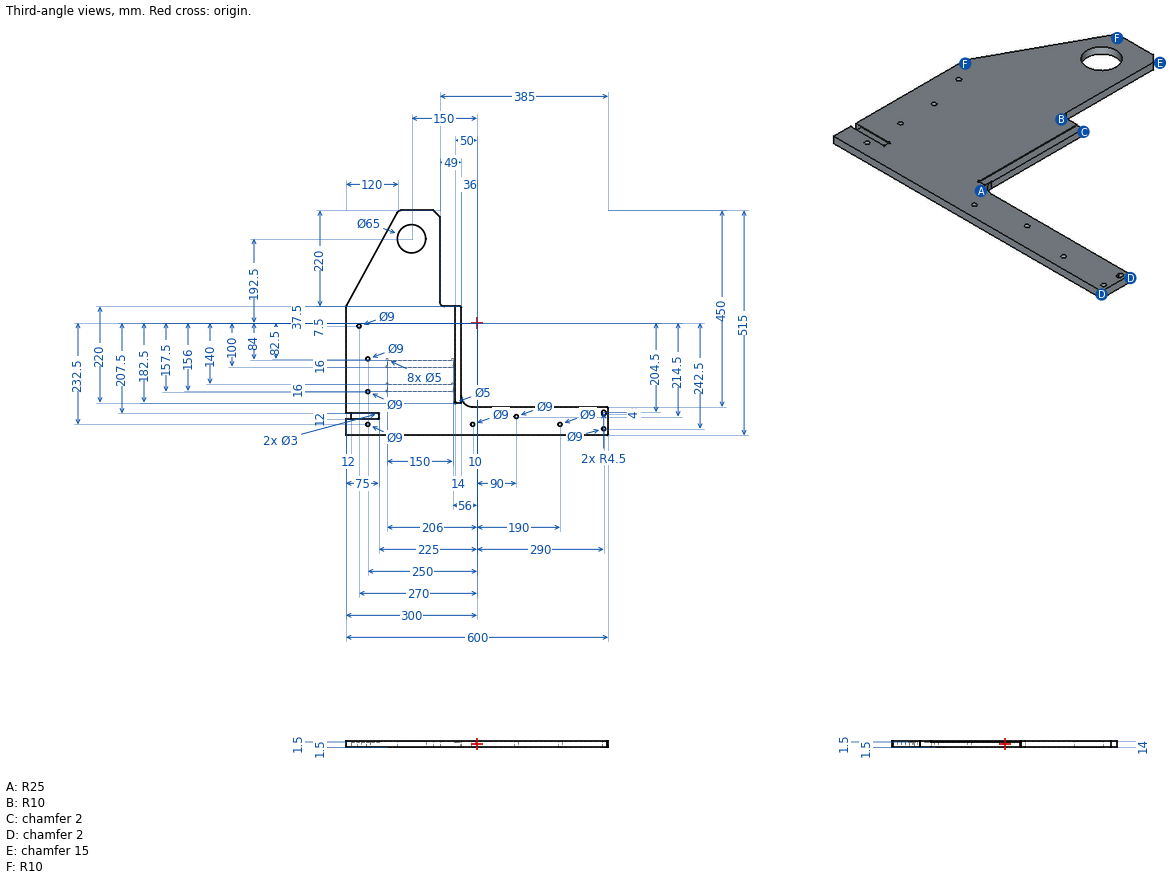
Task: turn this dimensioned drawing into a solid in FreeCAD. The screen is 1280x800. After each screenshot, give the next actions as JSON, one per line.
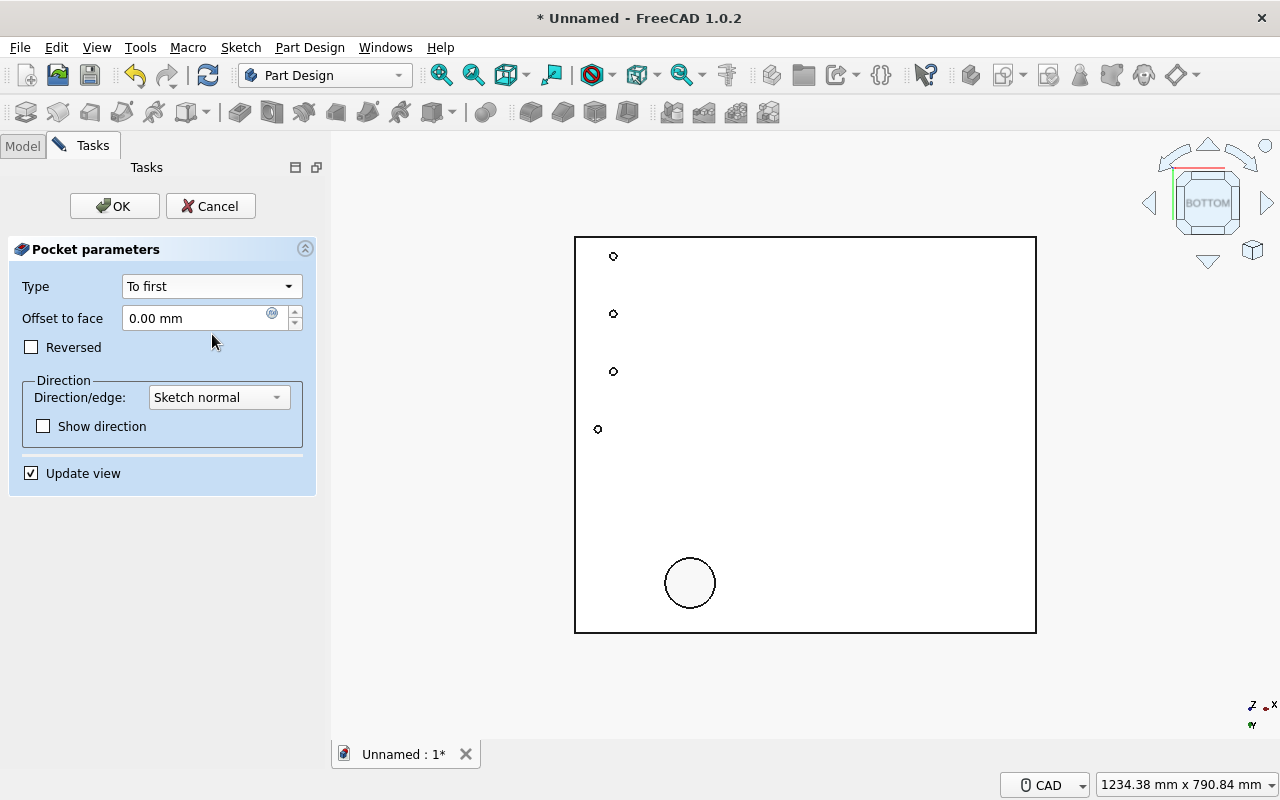
{"action": "left_click", "coordinate": [115, 206]}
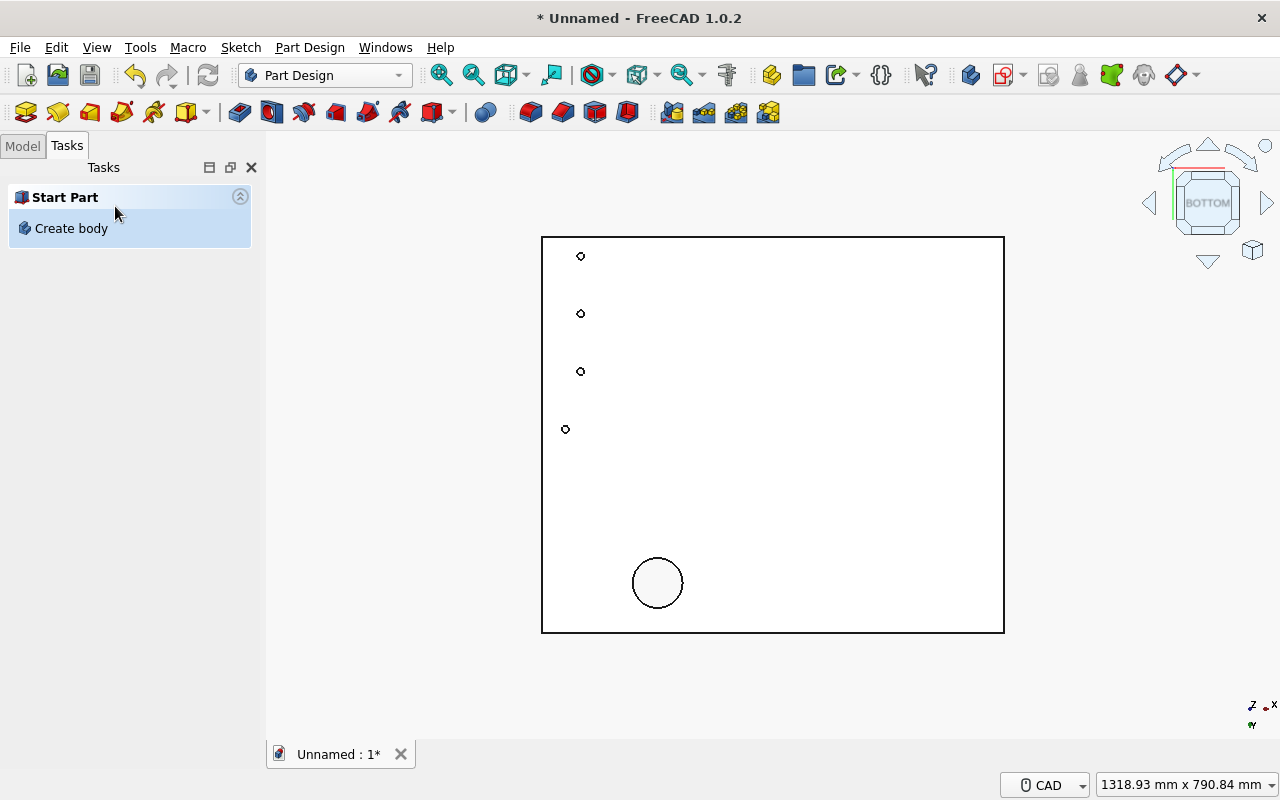
{"action": "left_click", "coordinate": [839, 434]}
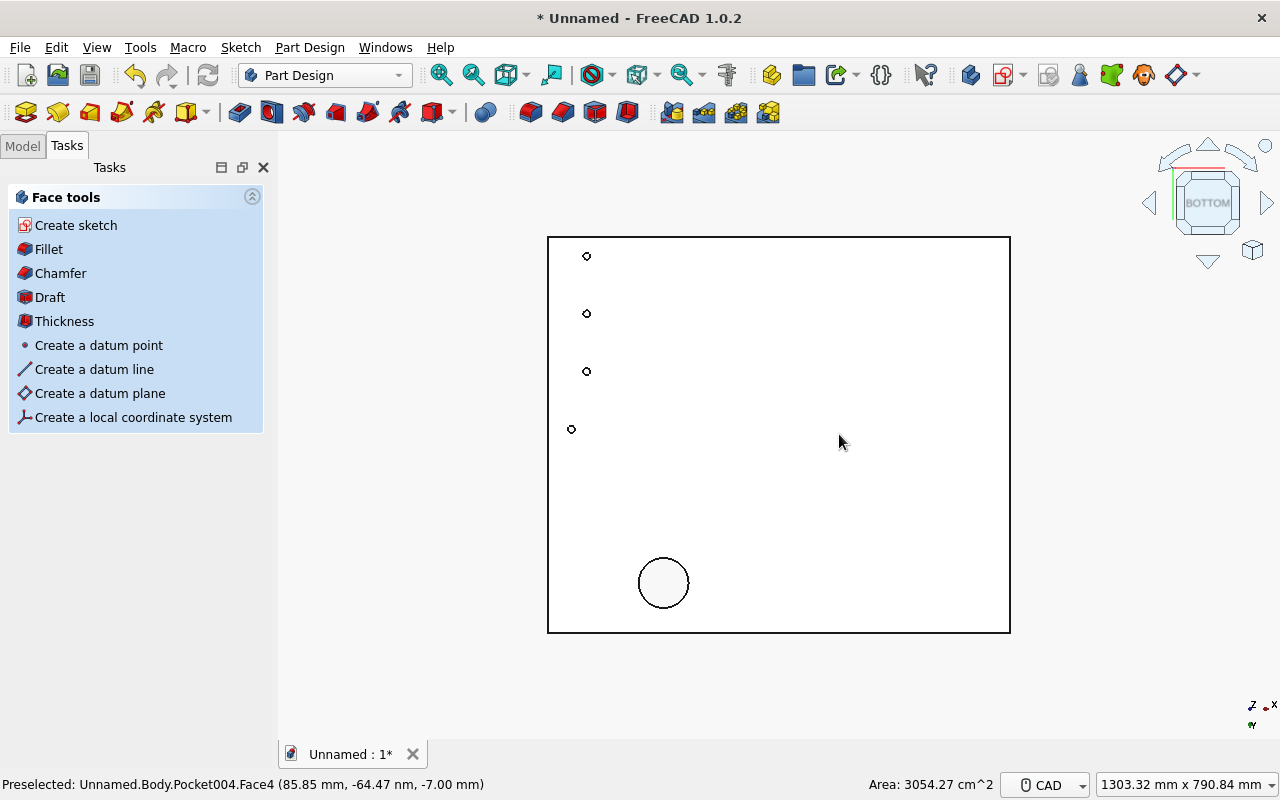
{"action": "left_click", "coordinate": [1004, 76]}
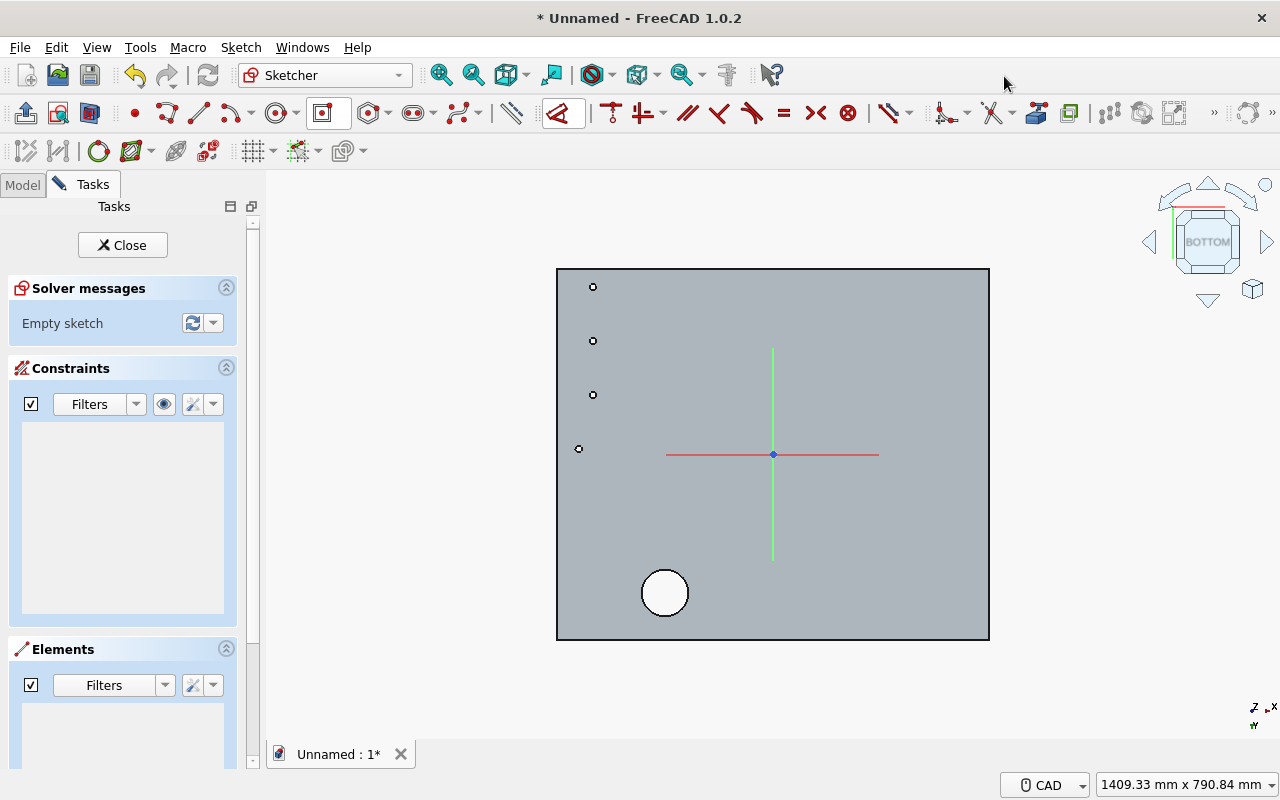
{"action": "scroll", "coordinate": [769, 278], "scroll_direction": "up", "scroll_amount": 15}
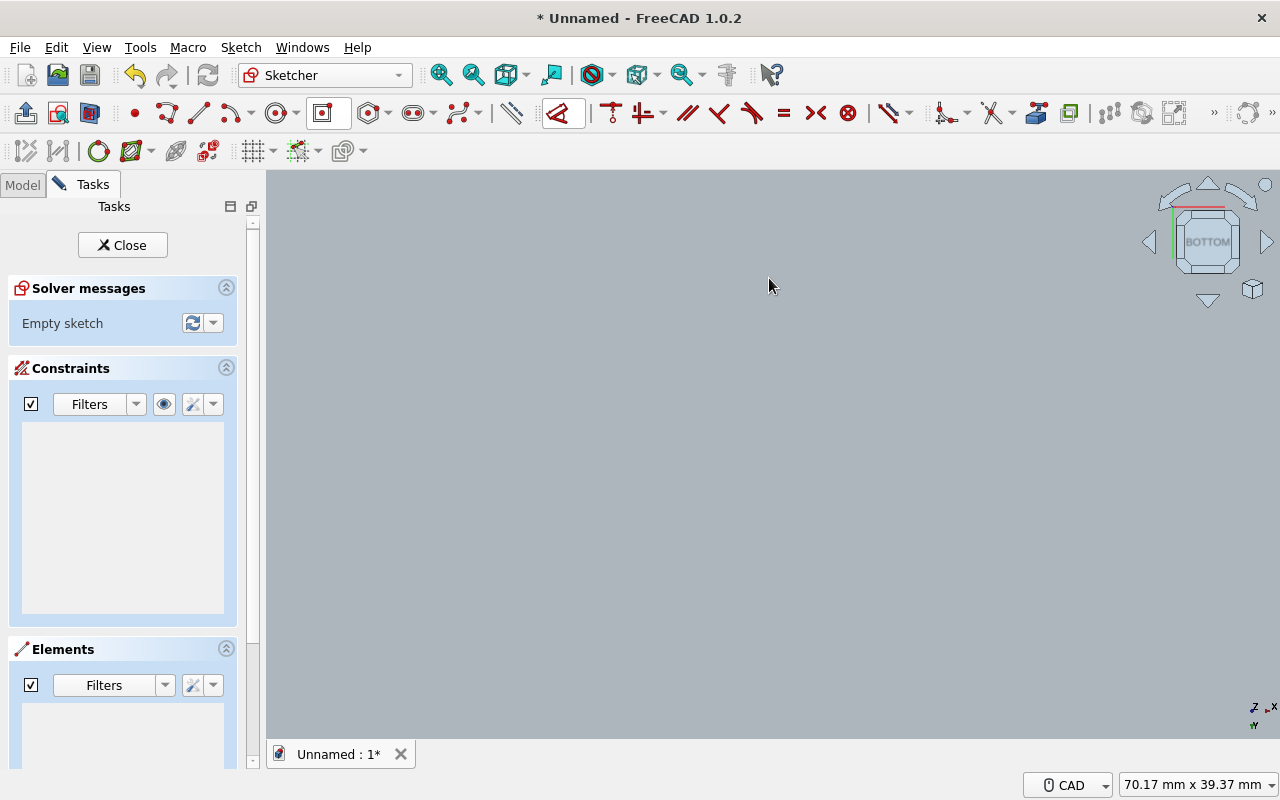
{"action": "scroll", "coordinate": [690, 462], "scroll_direction": "up", "scroll_amount": 5}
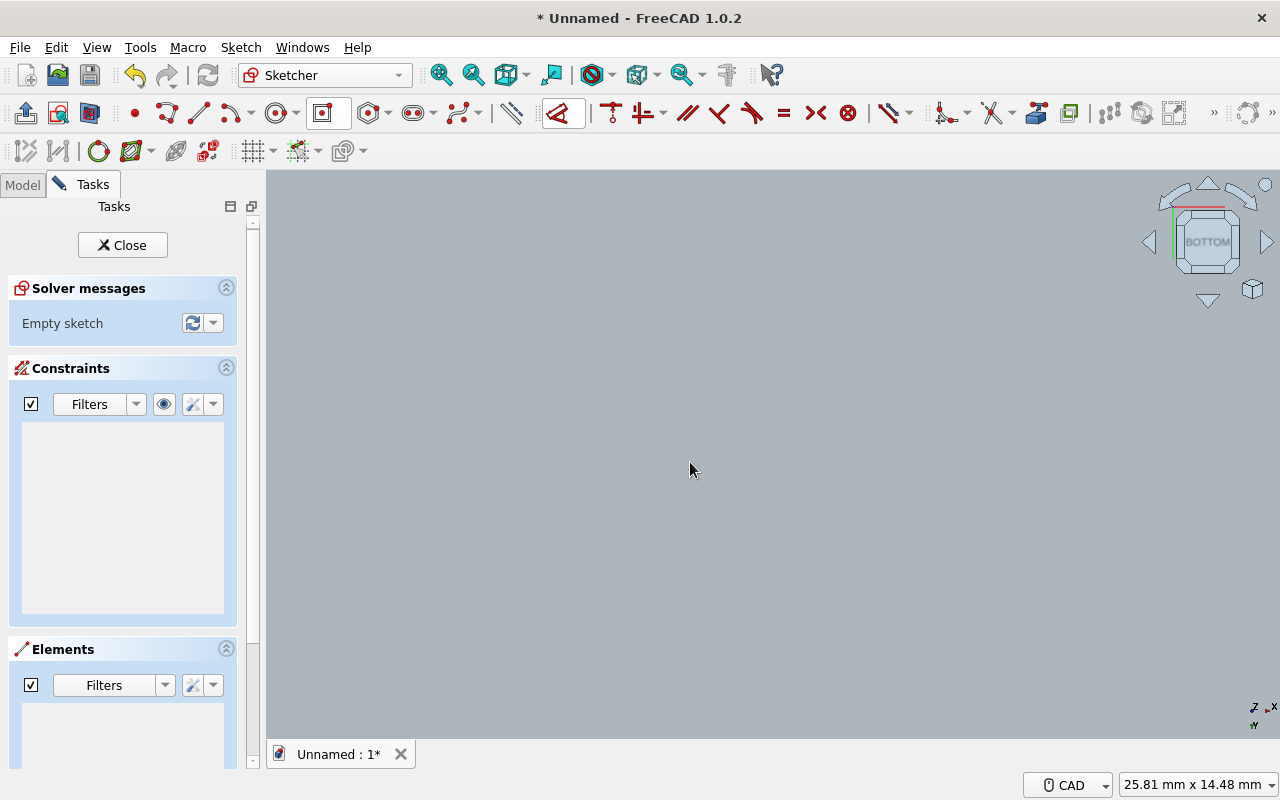
{"action": "left_click", "coordinate": [276, 114]}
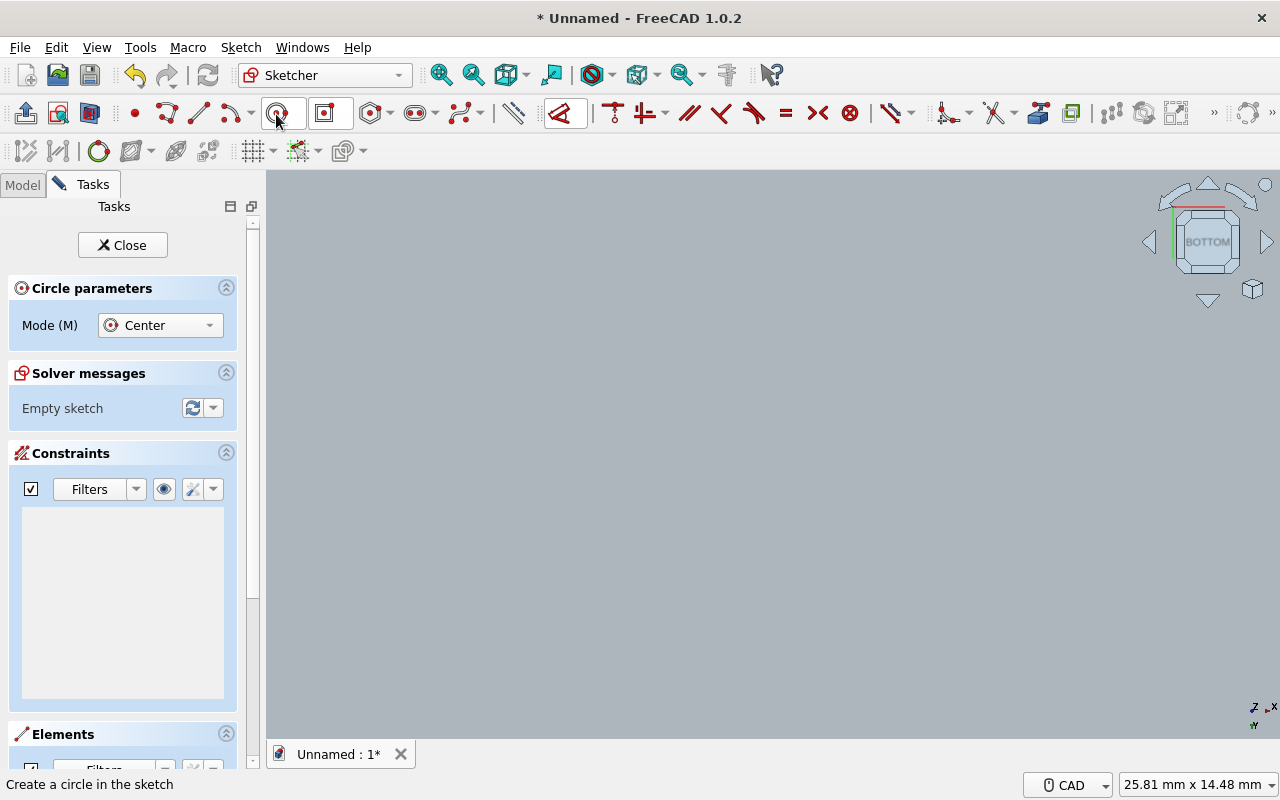
{"action": "left_click", "coordinate": [704, 454]}
{"action": "mouse_move", "coordinate": [829, 329]}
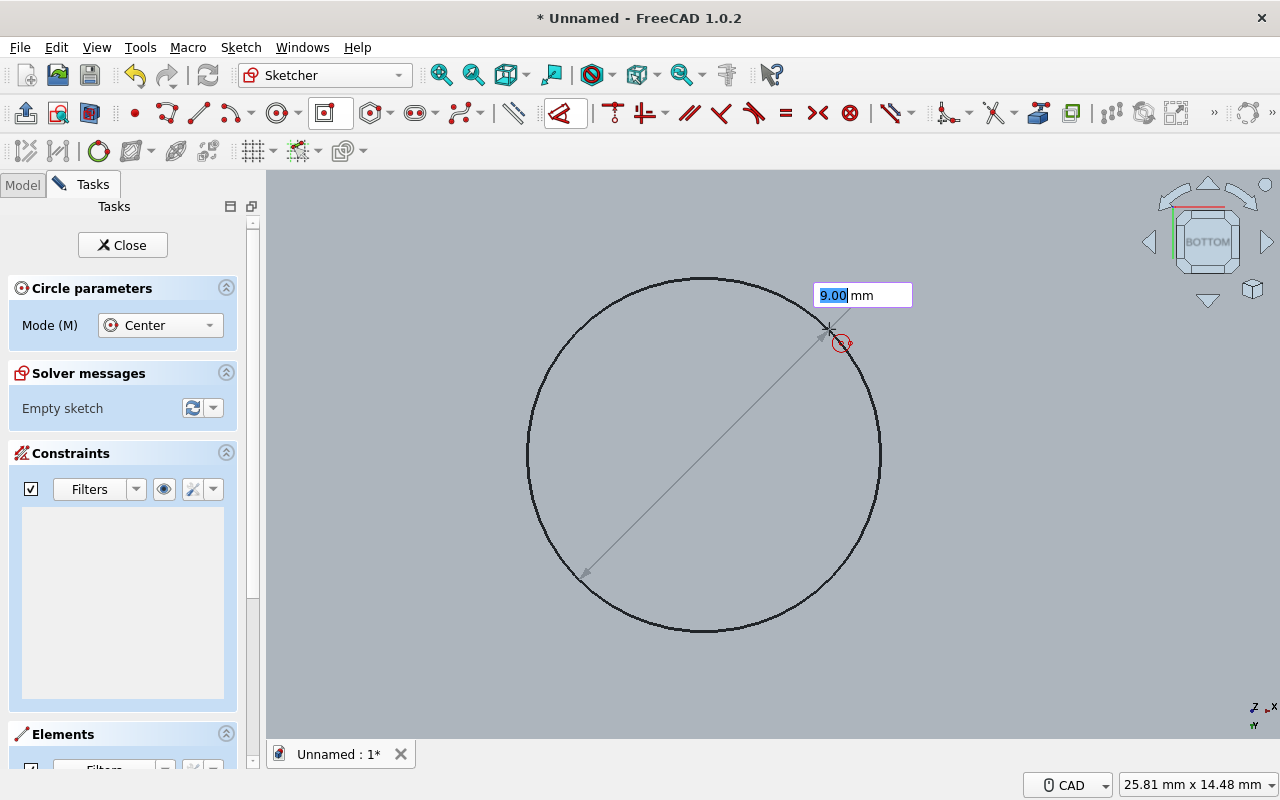
{"action": "type", "text": "9"}
{"action": "key", "text": "Return"}
{"action": "key", "text": "Escape"}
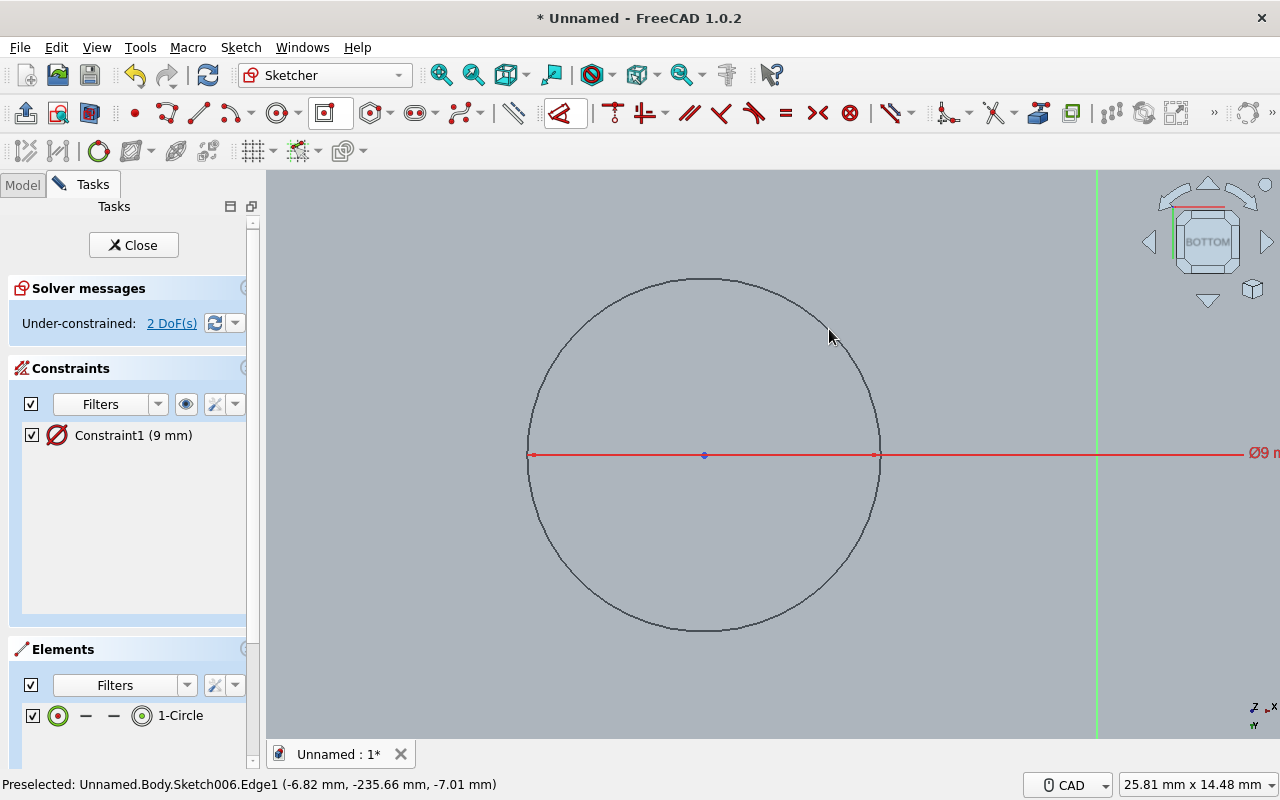
{"action": "left_click", "coordinate": [704, 455]}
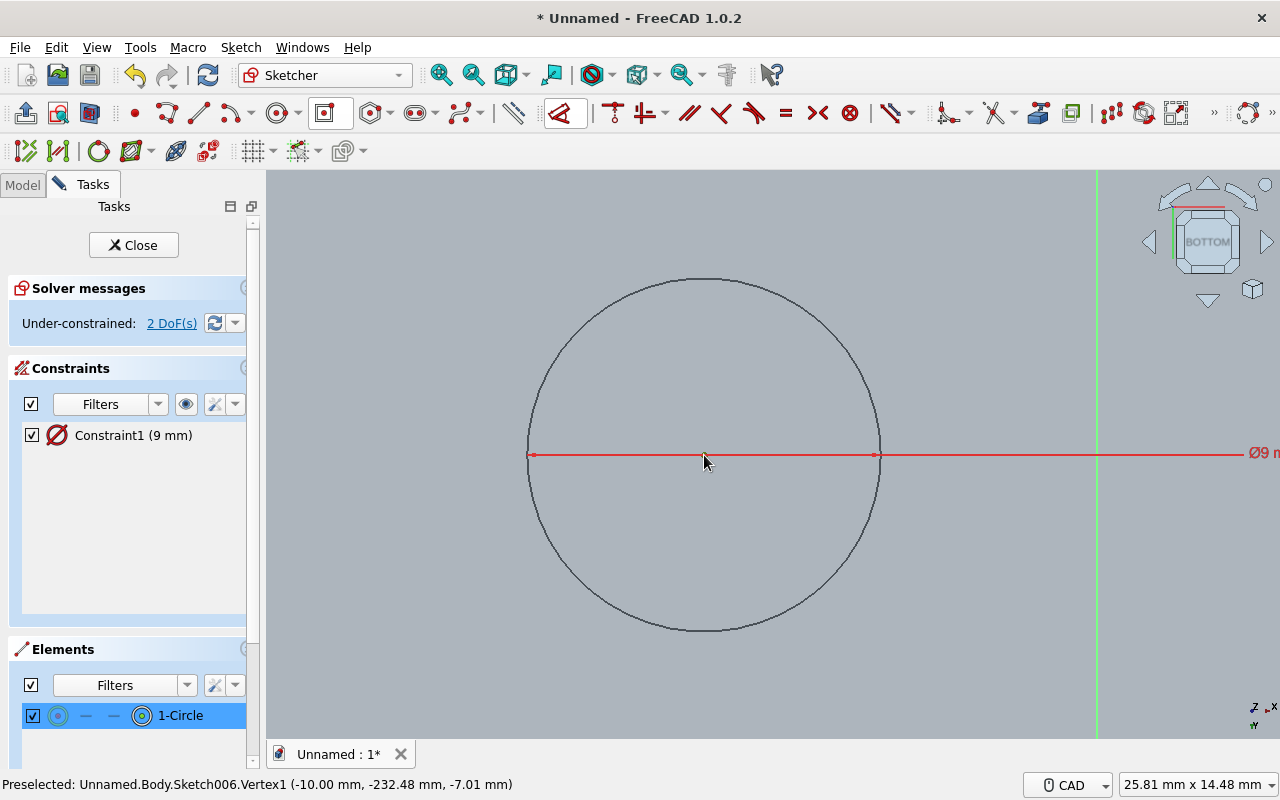
{"action": "key", "text": "l"}